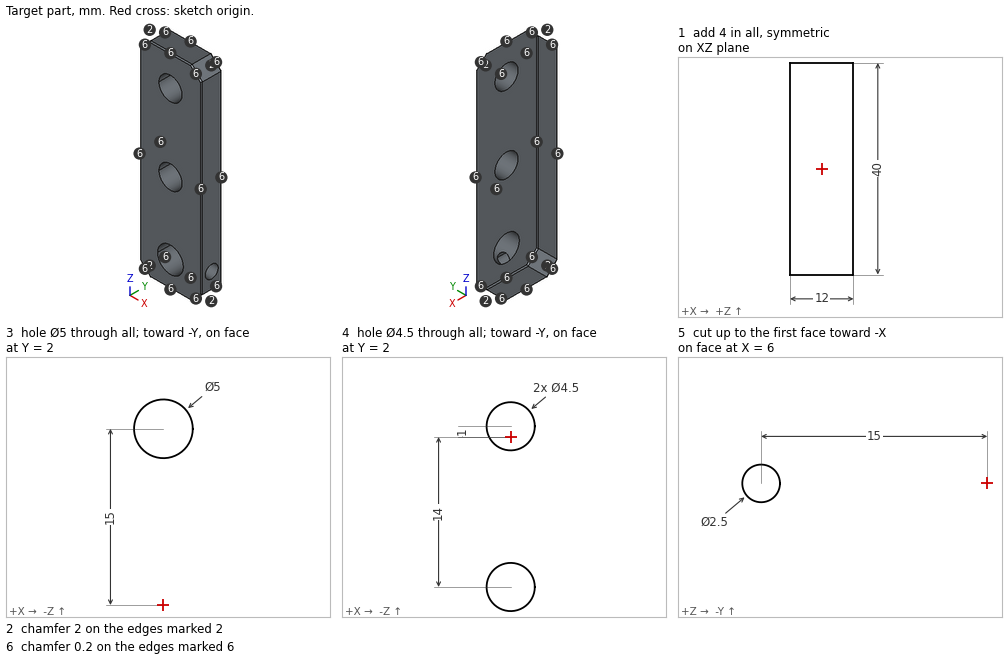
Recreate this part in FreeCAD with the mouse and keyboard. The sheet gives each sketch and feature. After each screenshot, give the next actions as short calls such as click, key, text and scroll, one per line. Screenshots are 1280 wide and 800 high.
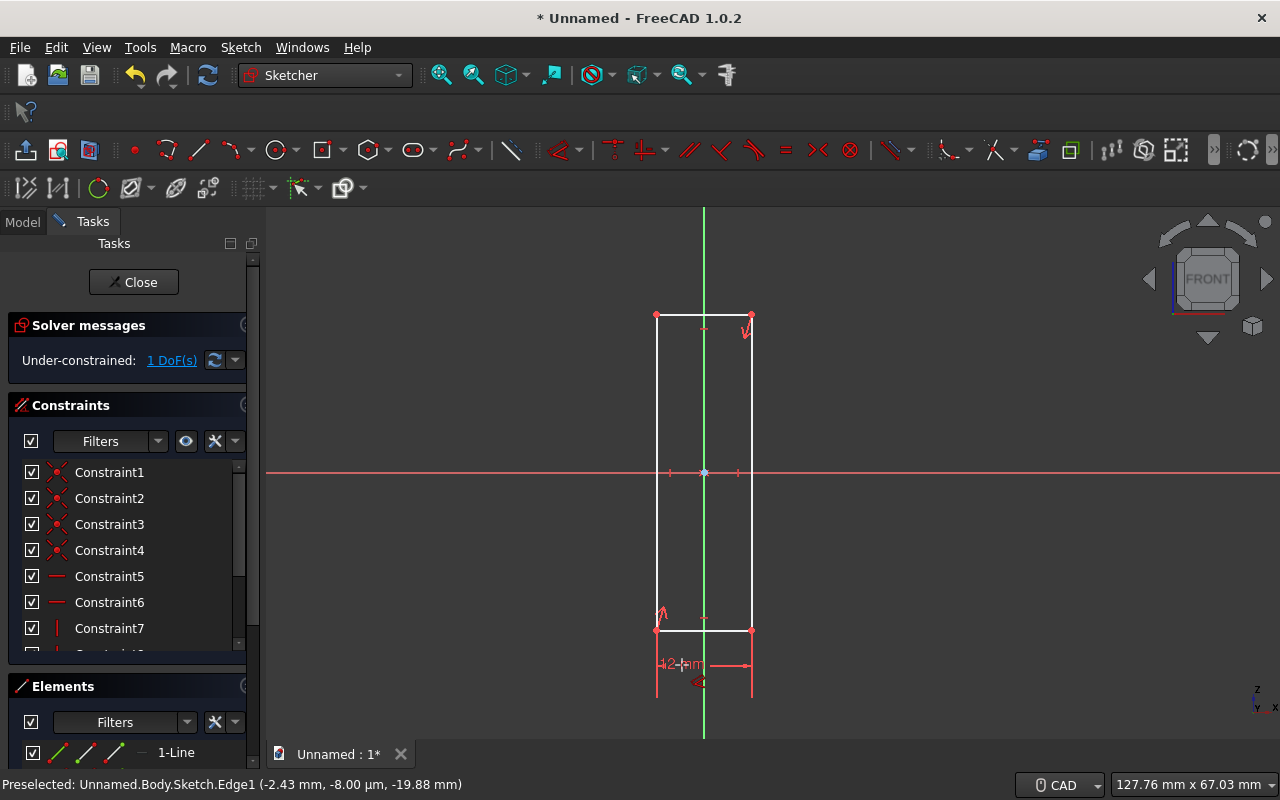
click(752, 536)
click(786, 400)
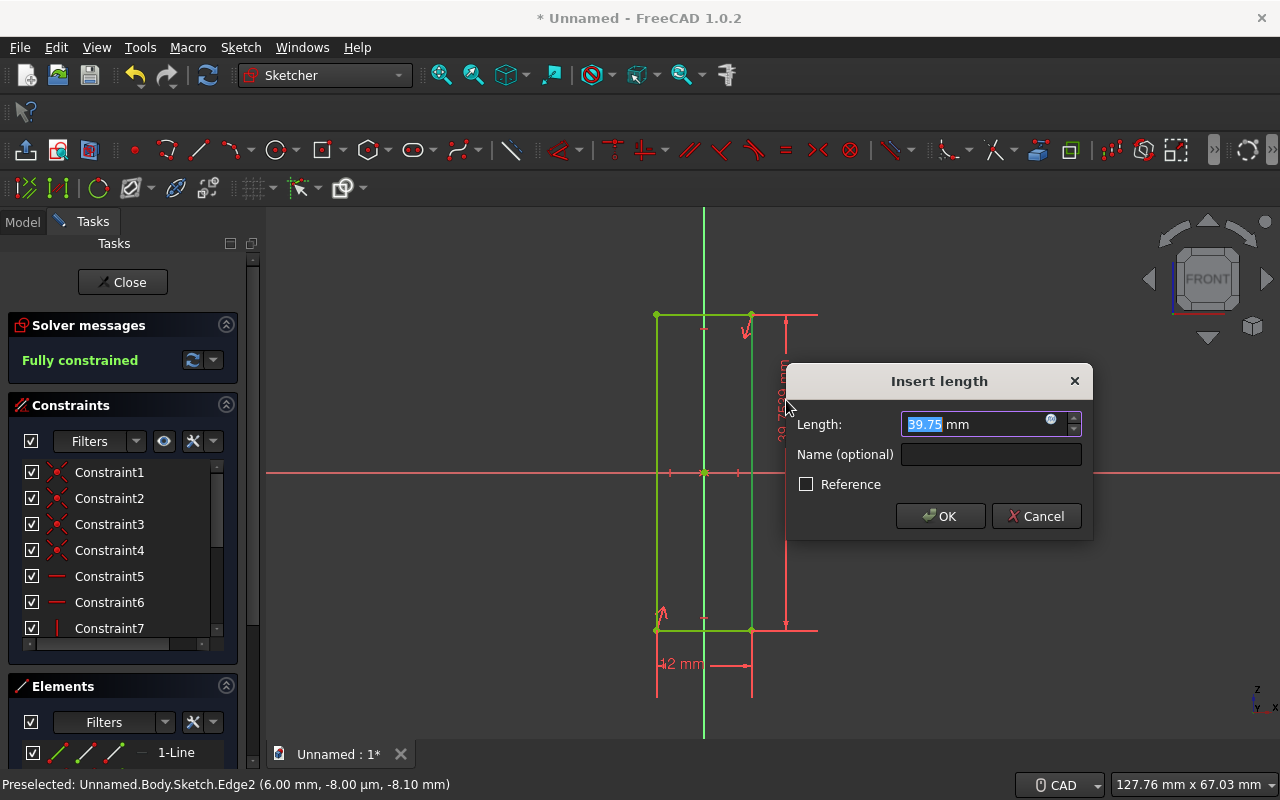
text(40)
key(Return)
key(Escape)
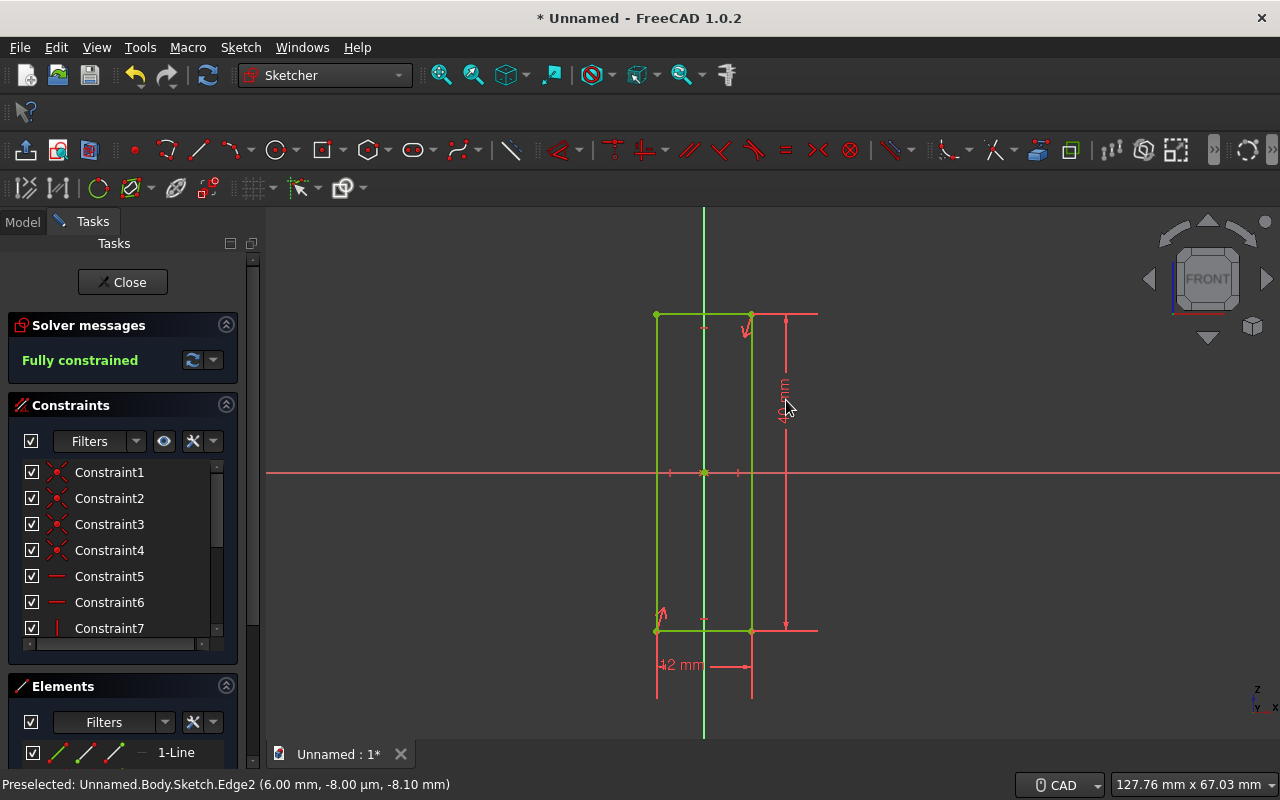
click(123, 282)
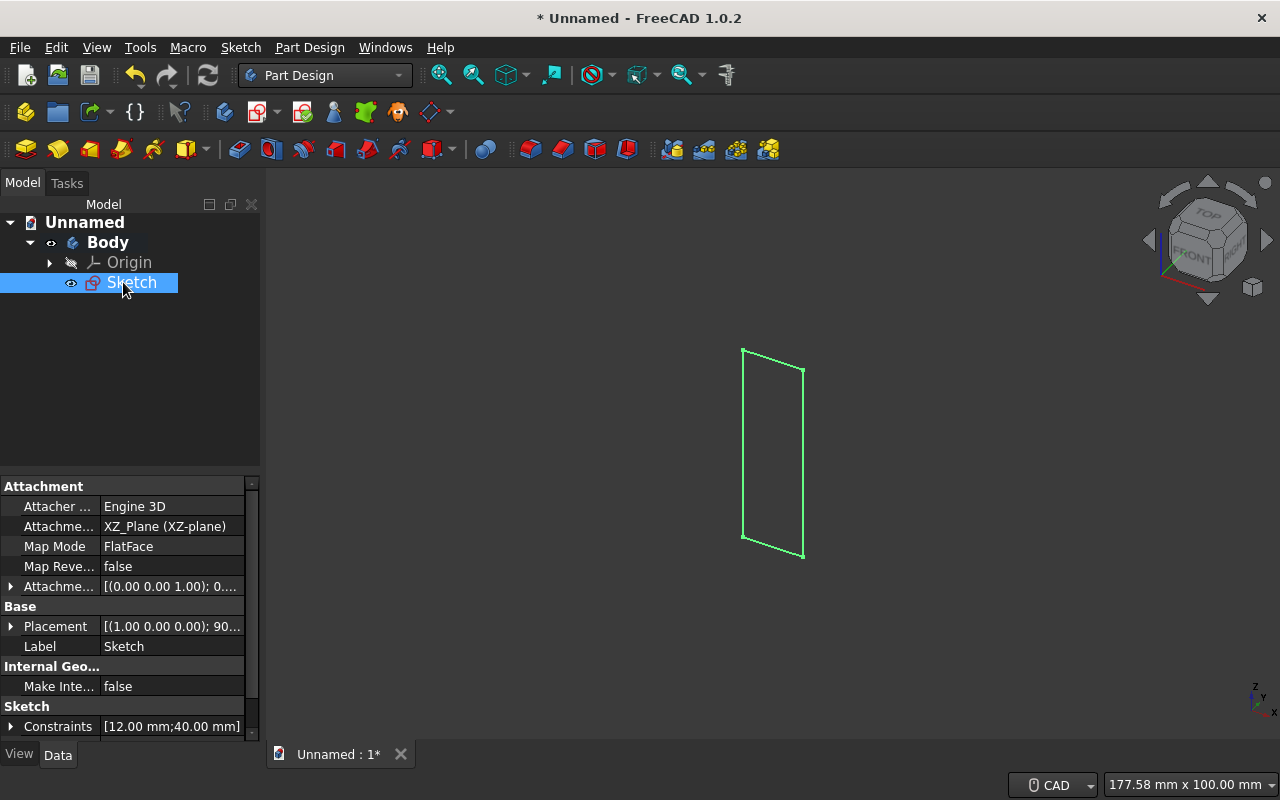
click(26, 150)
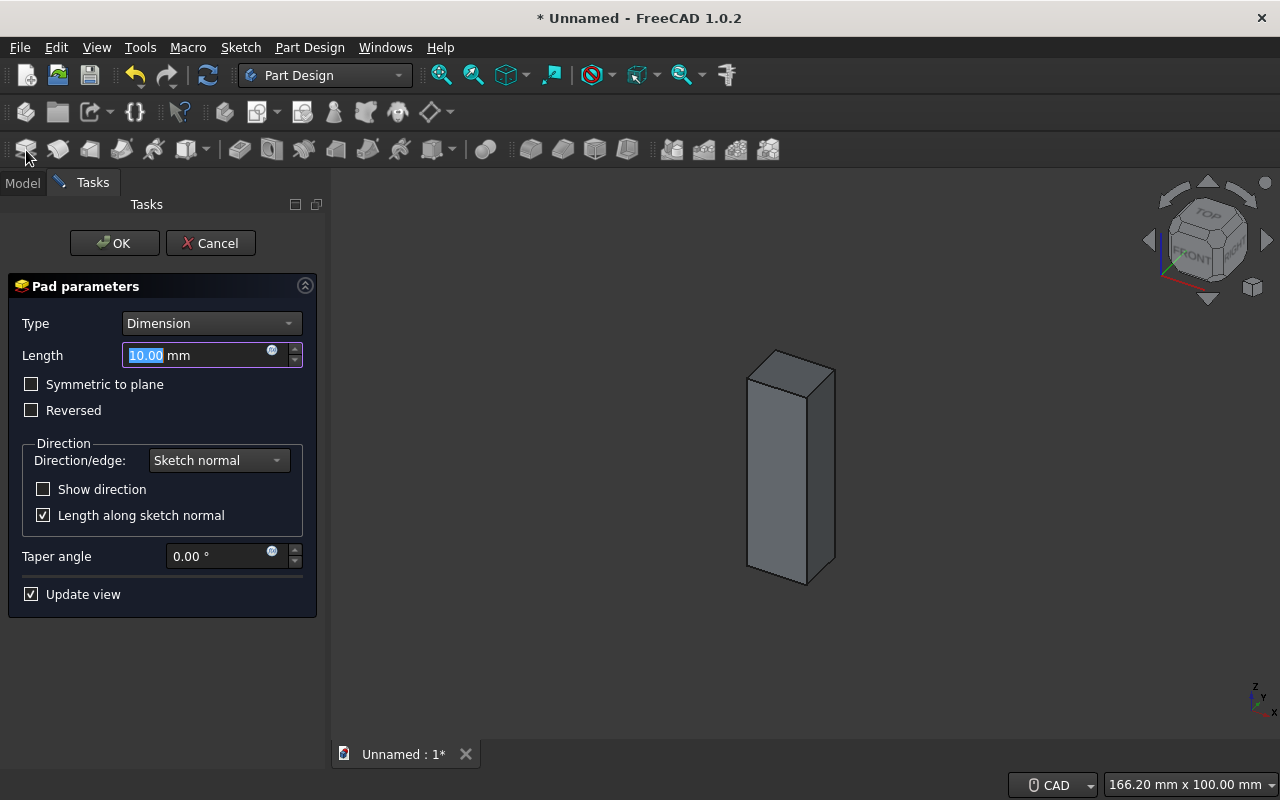
text(4)
key(Tab)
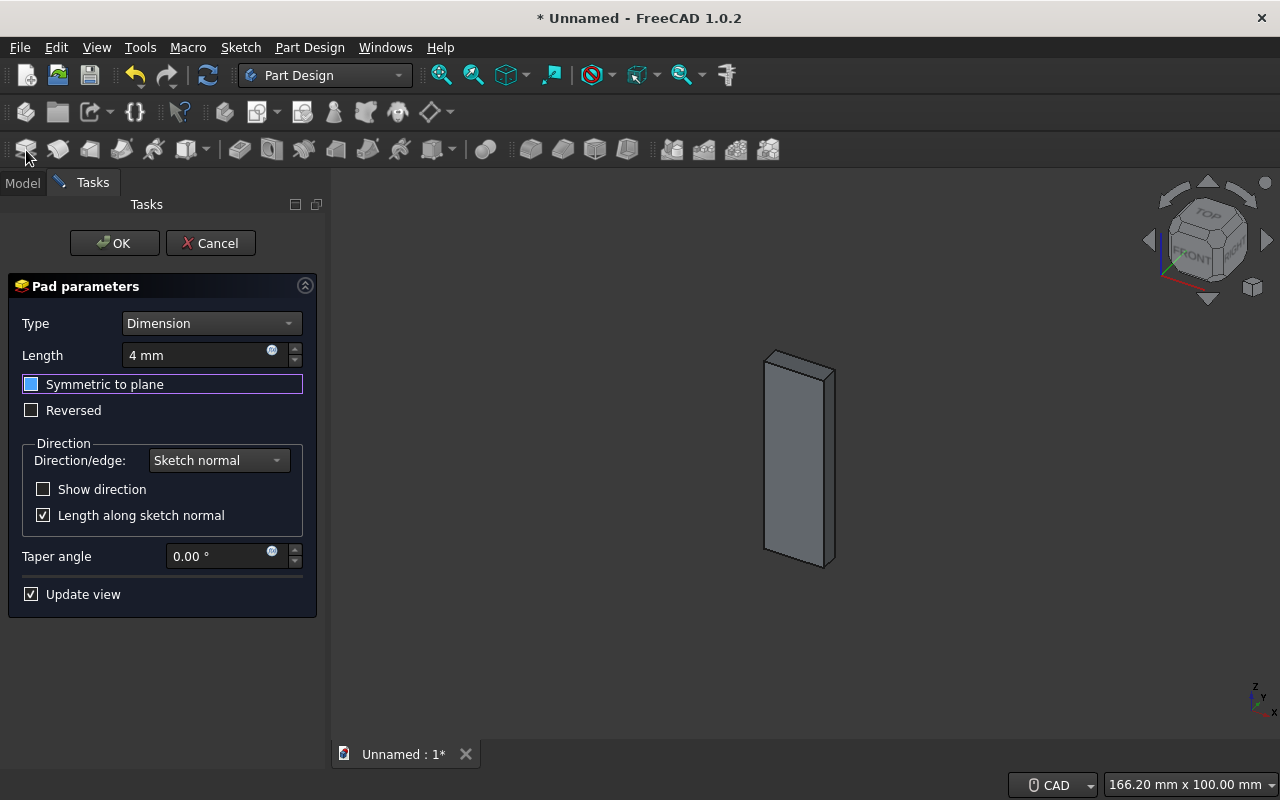
click(30, 384)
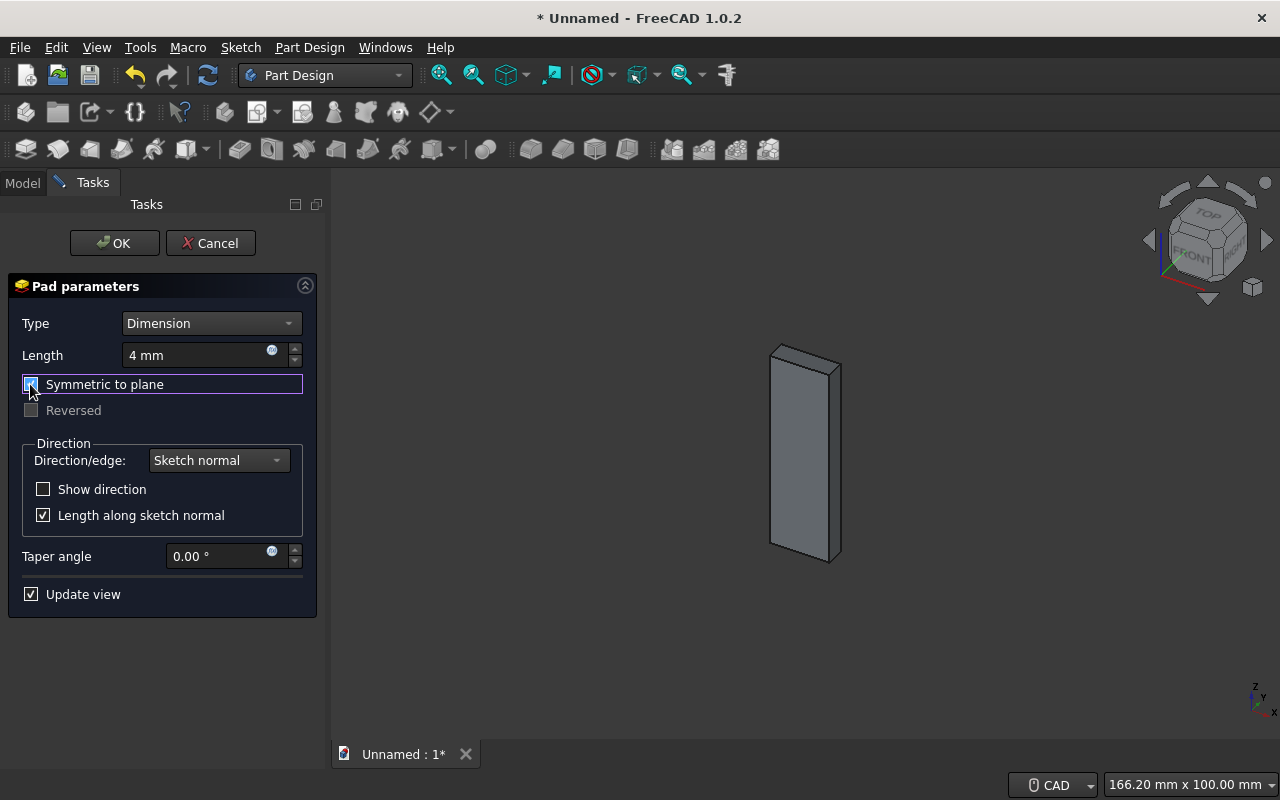
click(115, 243)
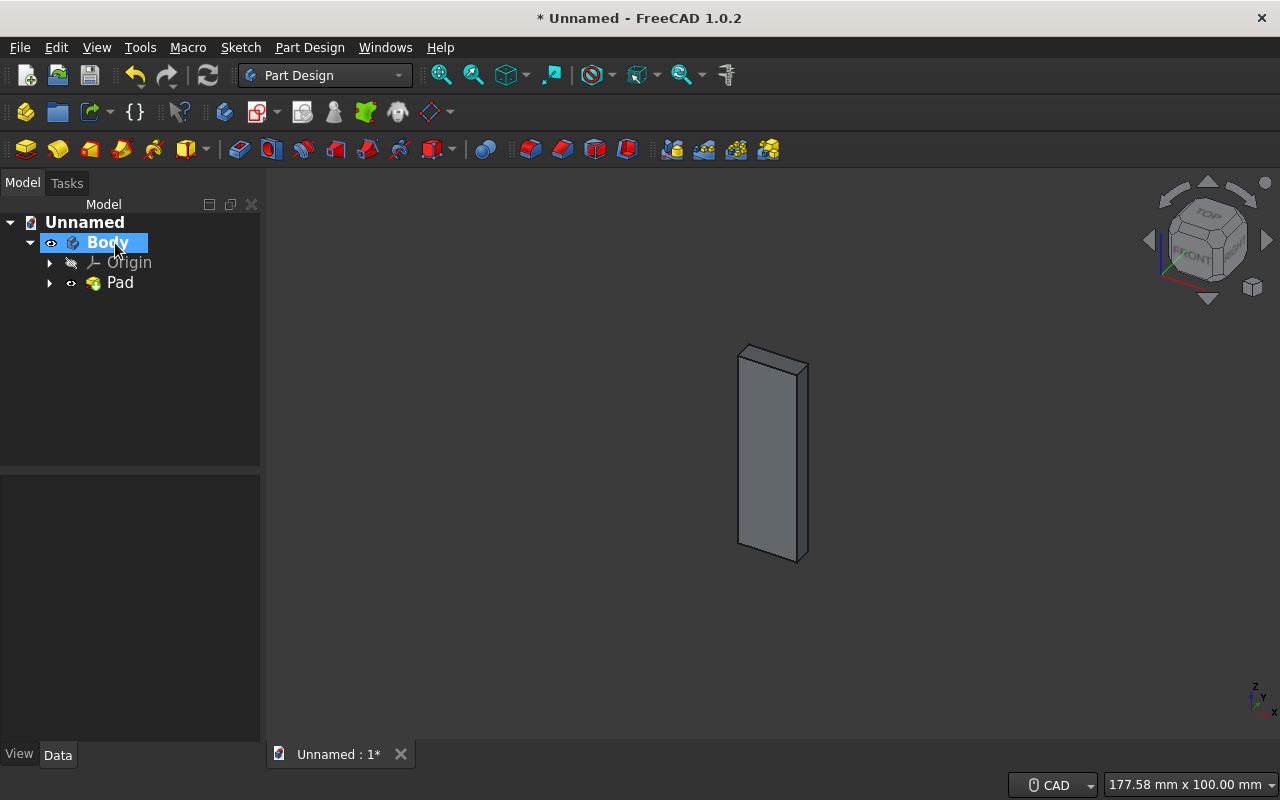
click(442, 76)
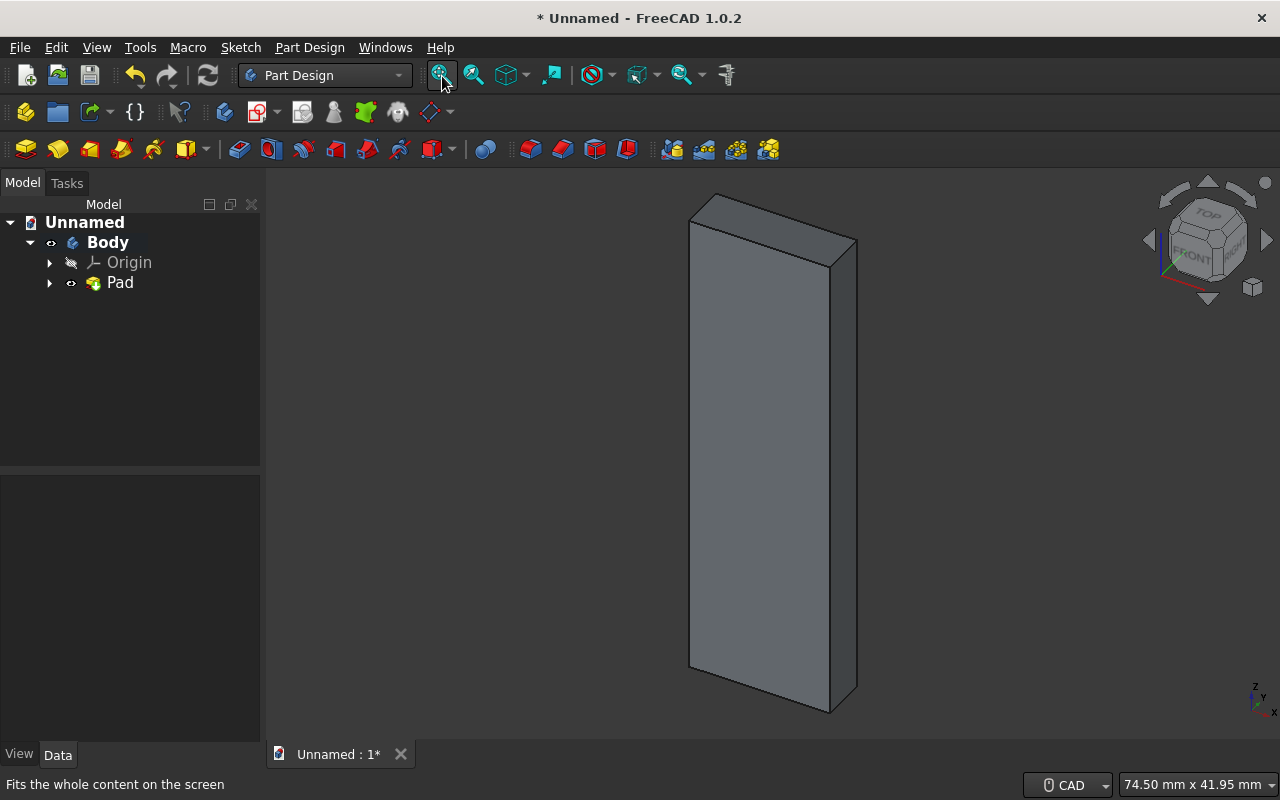
click(844, 253)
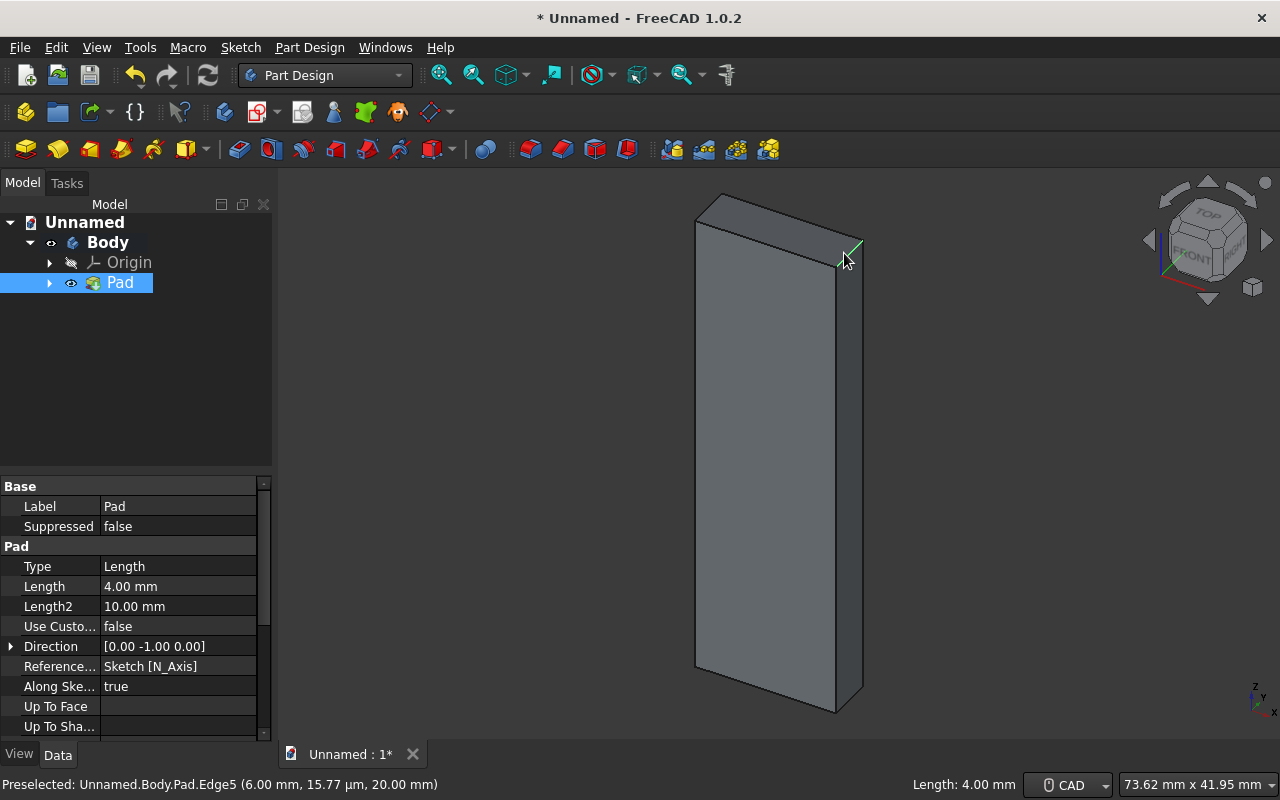
key(0)